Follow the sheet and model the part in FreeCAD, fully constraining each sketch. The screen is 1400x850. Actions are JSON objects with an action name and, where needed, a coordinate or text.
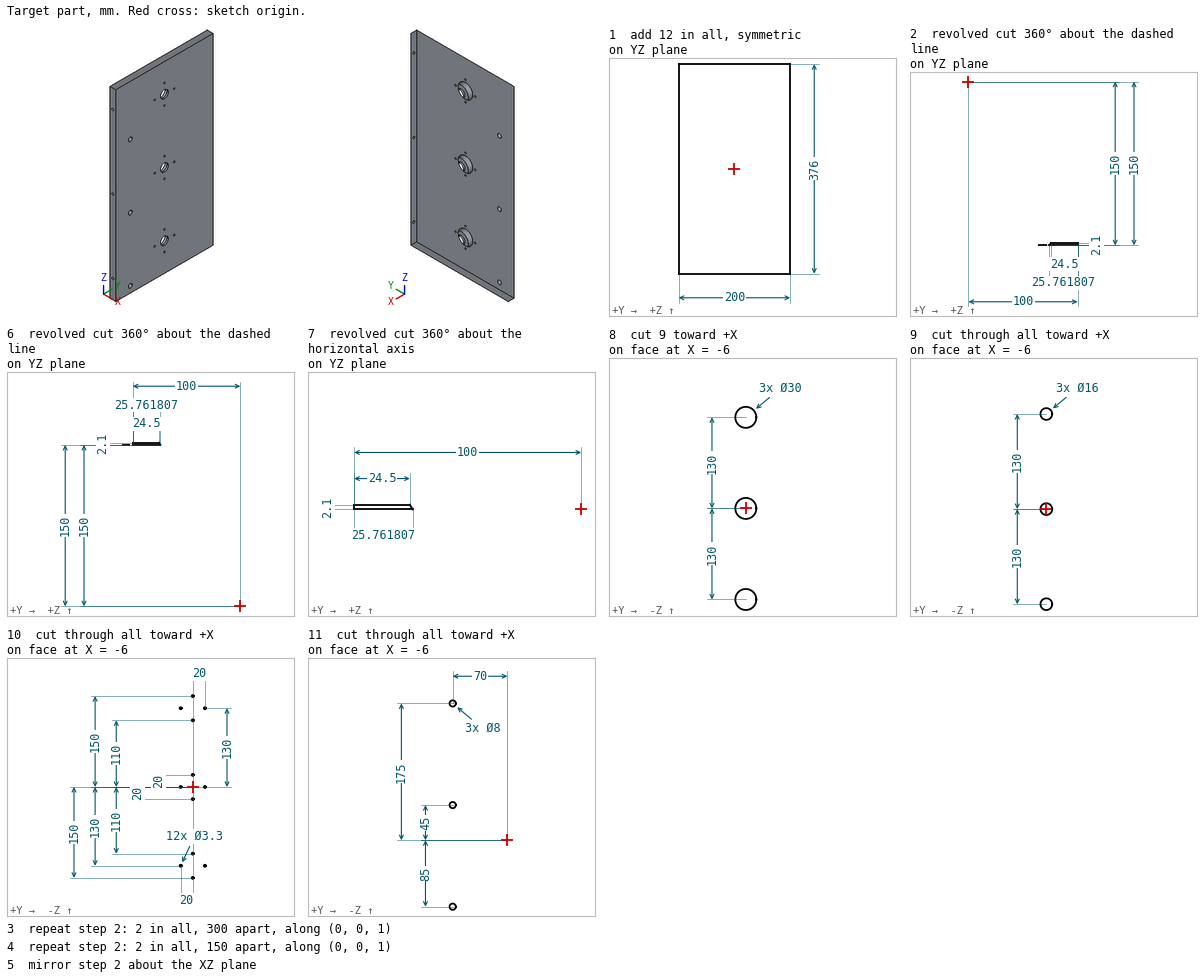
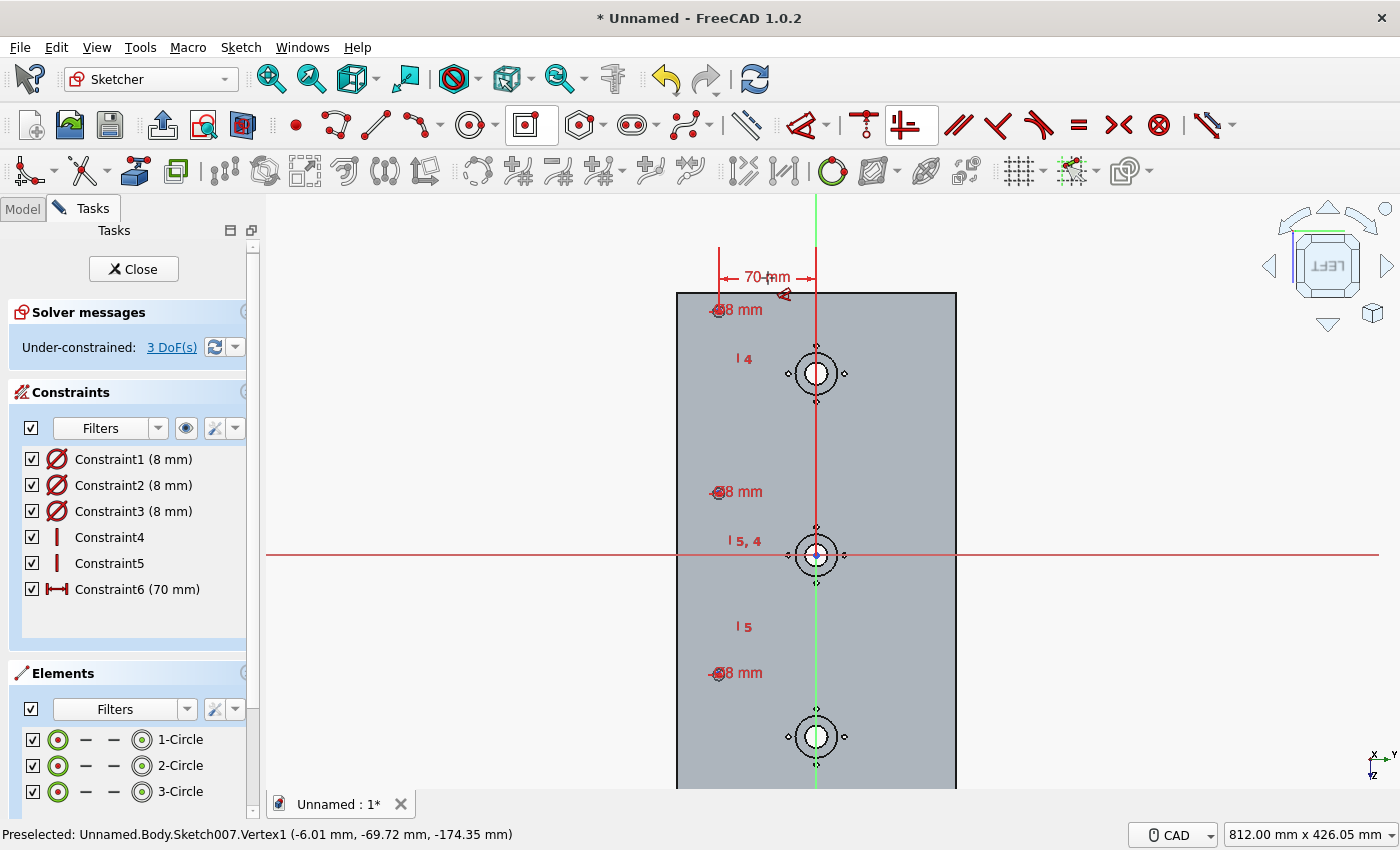
{"action": "left_click", "coordinate": [719, 494]}
{"action": "left_click", "coordinate": [850, 525]}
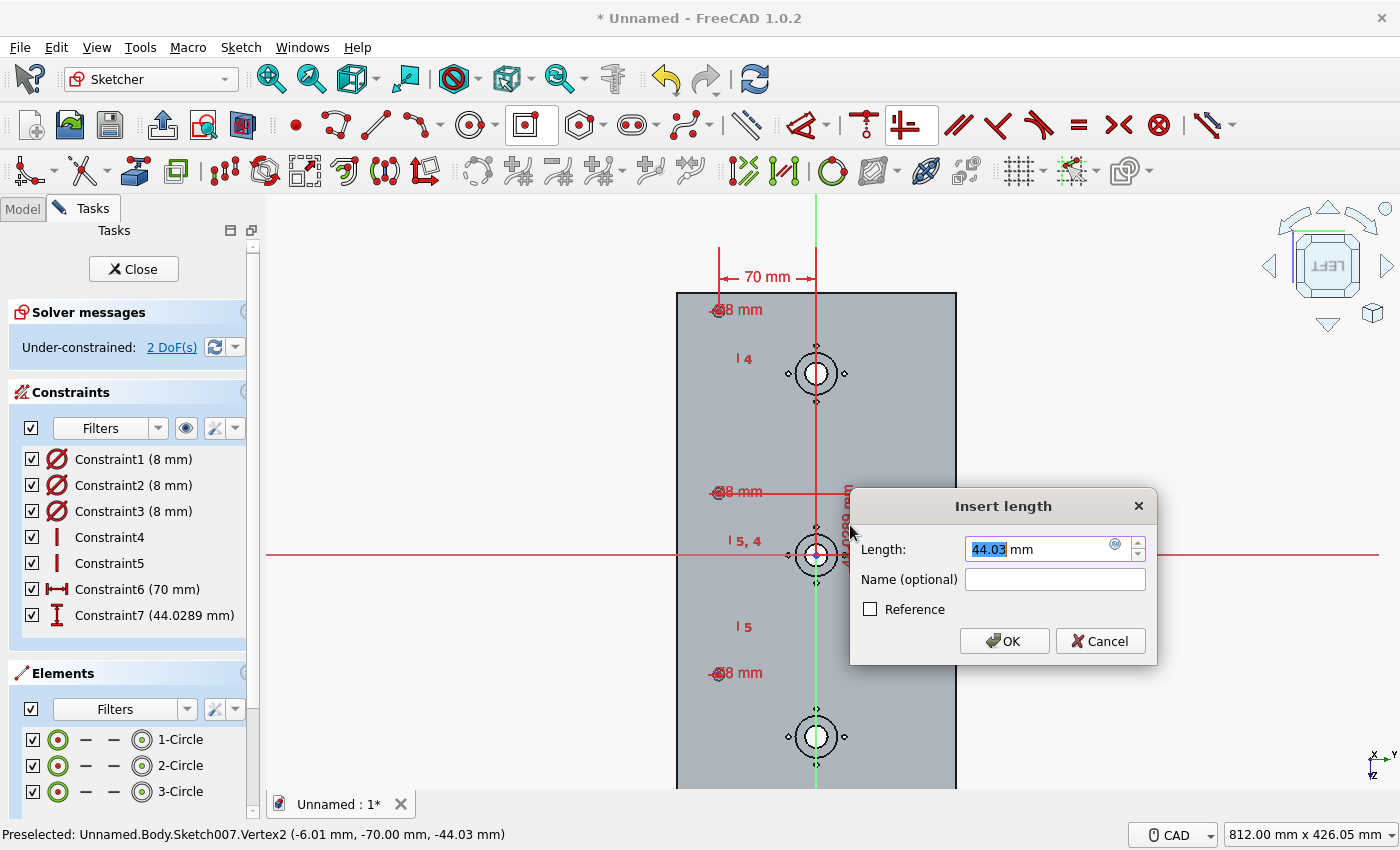
{"action": "type", "text": "45"}
{"action": "key", "text": "Return"}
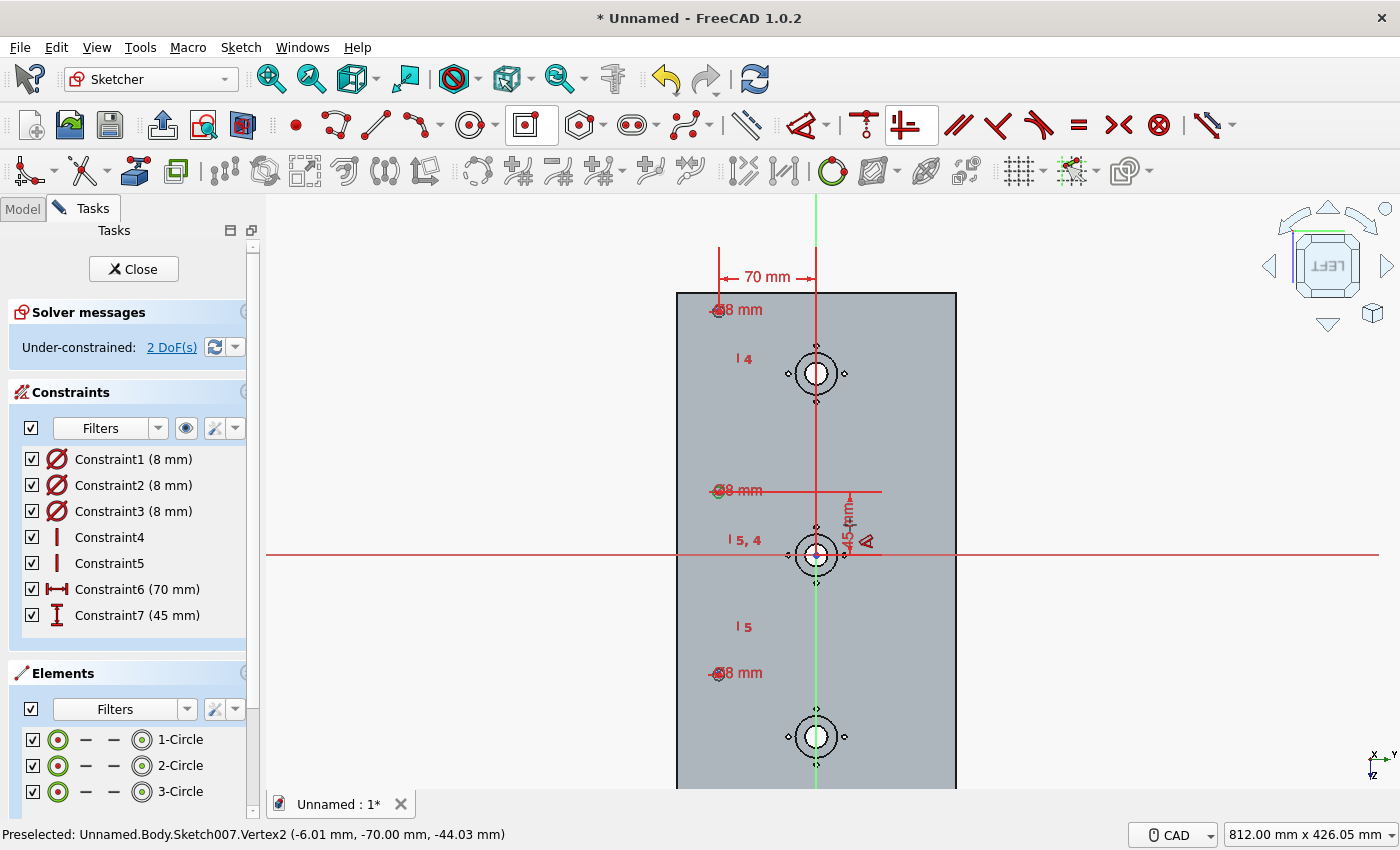
{"action": "left_click", "coordinate": [719, 675]}
{"action": "left_click", "coordinate": [850, 615]}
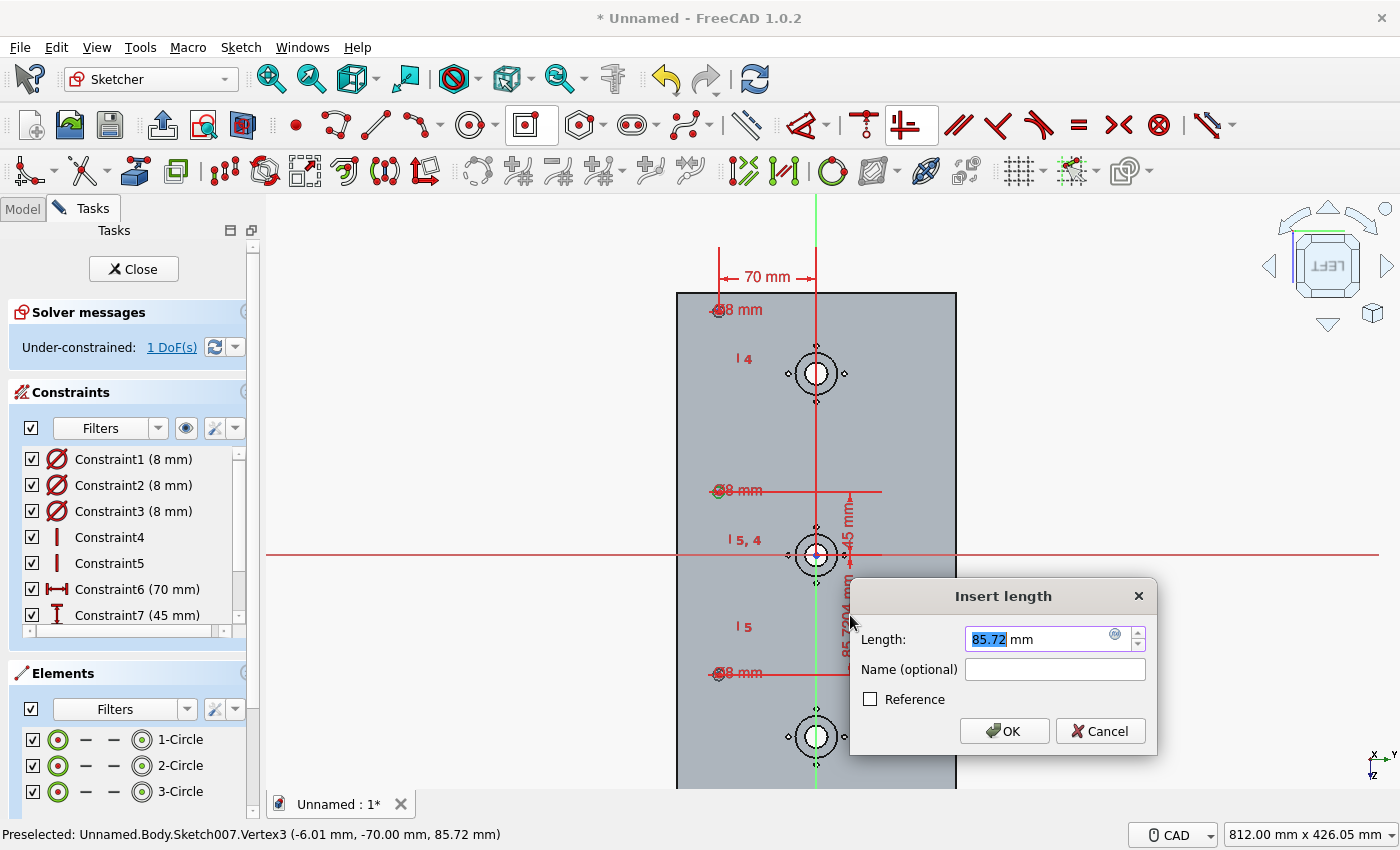
{"action": "type", "text": "85"}
{"action": "key", "text": "Return"}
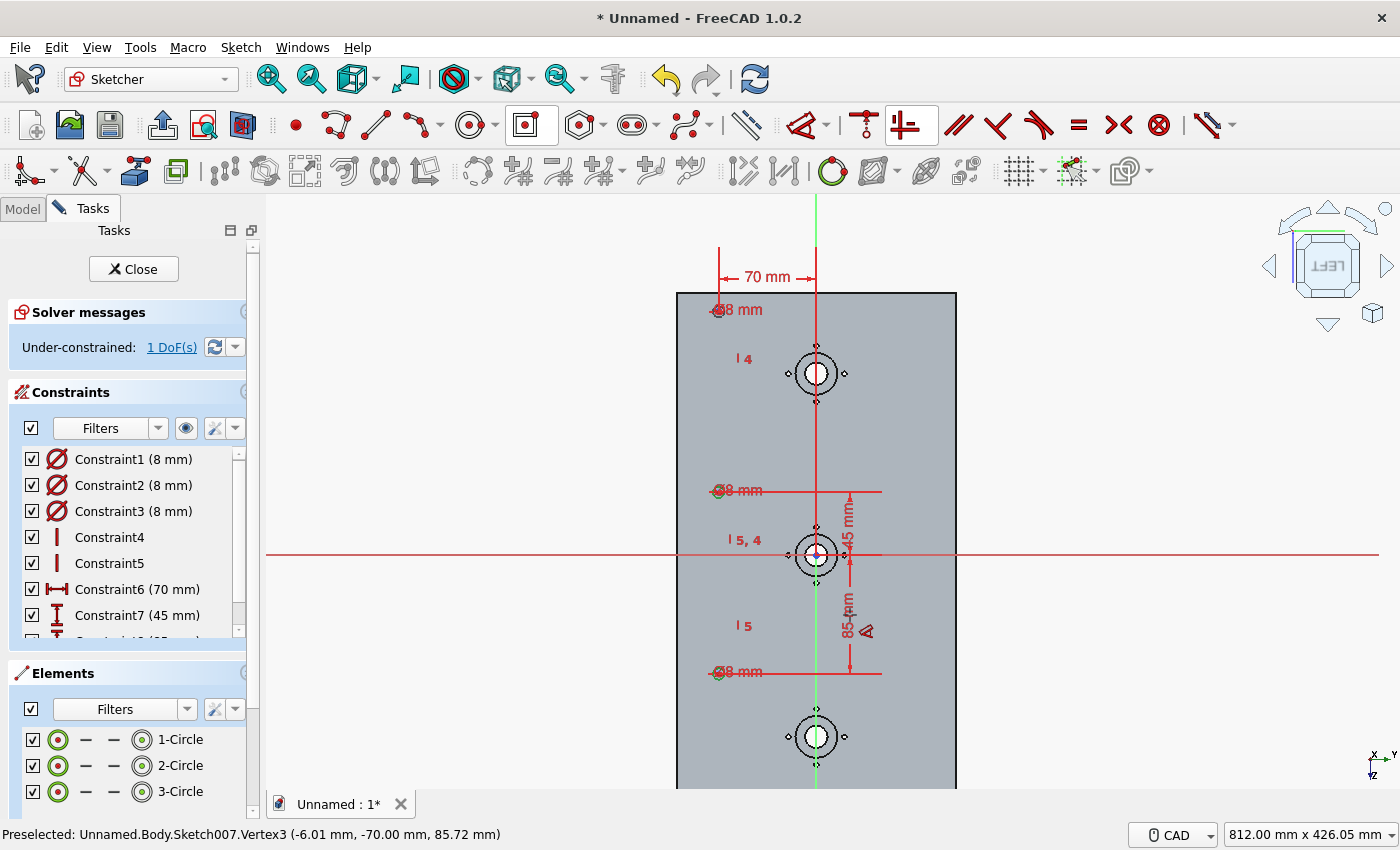
{"action": "left_click", "coordinate": [719, 312]}
{"action": "left_click", "coordinate": [850, 434]}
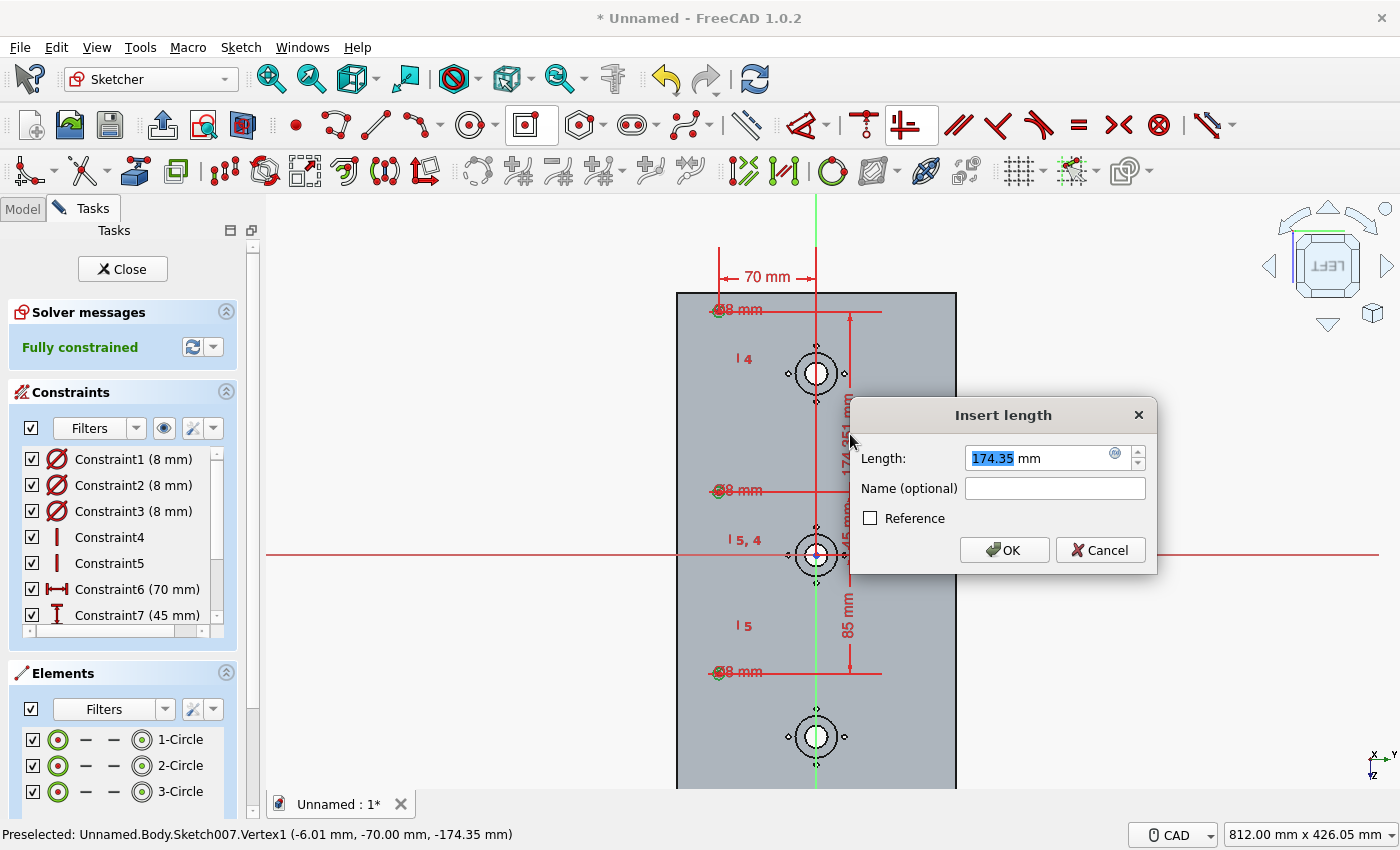
{"action": "type", "text": "175"}
{"action": "key", "text": "Return"}
{"action": "key", "text": "Escape"}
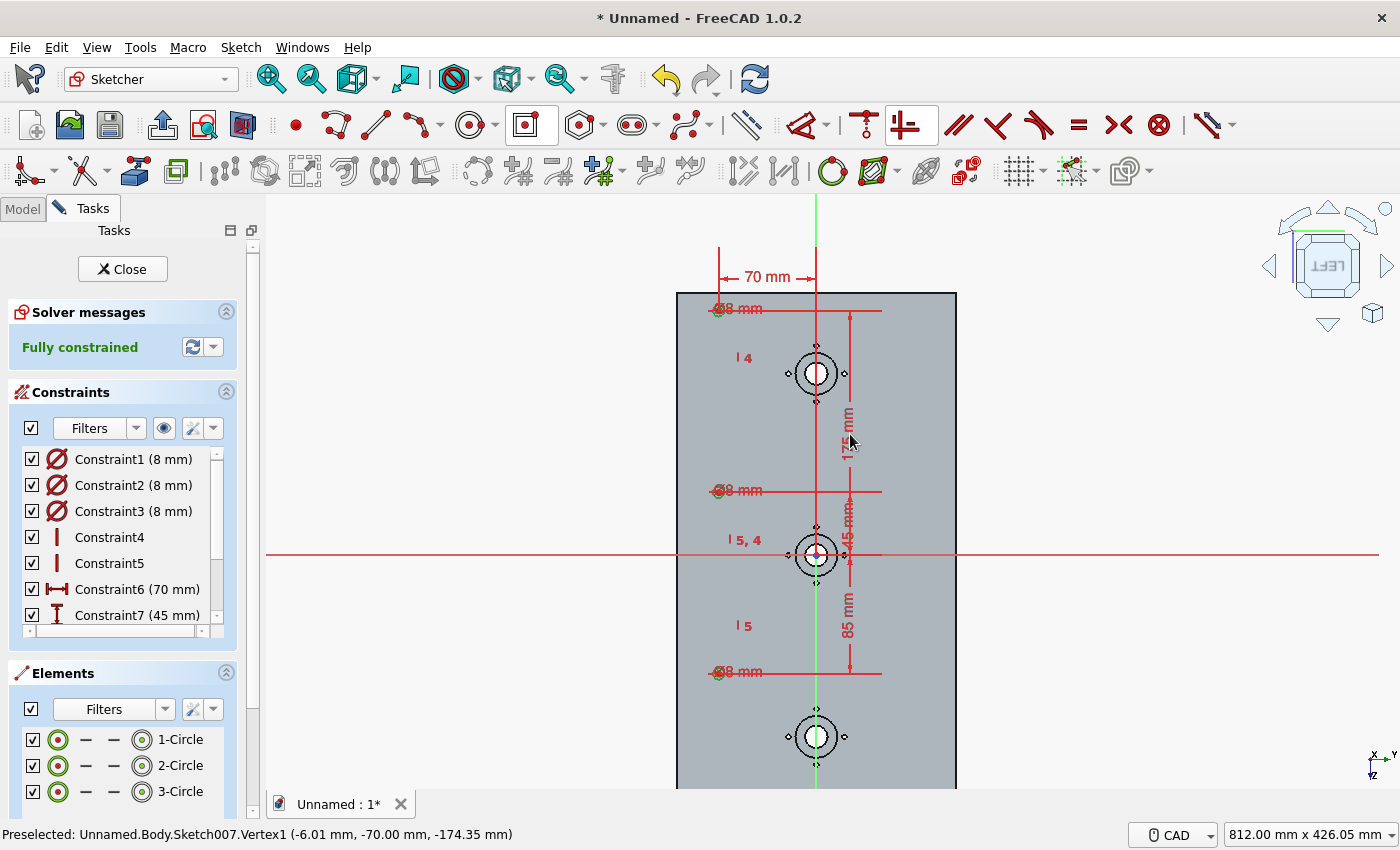
{"action": "left_click", "coordinate": [123, 269]}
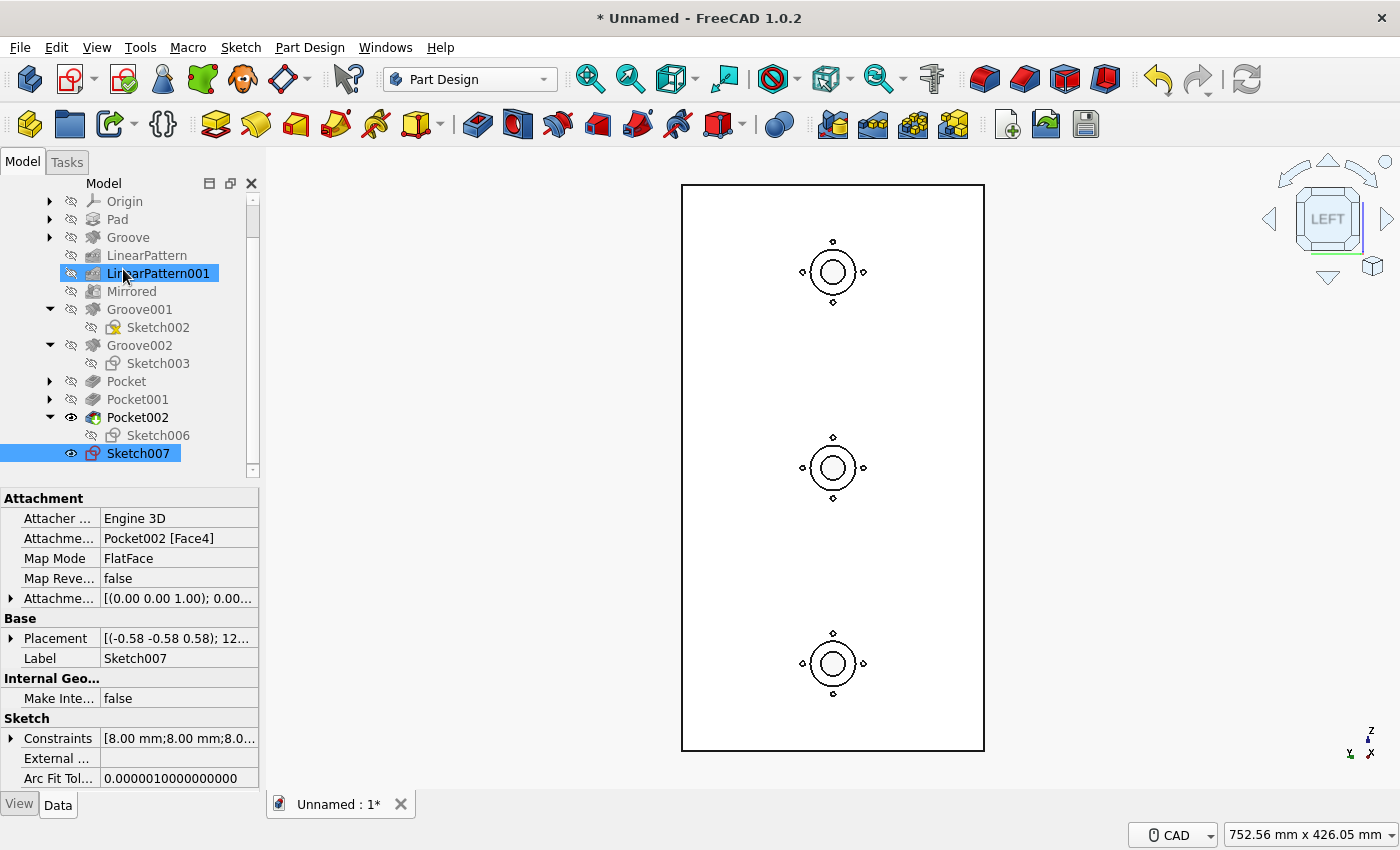
{"action": "left_click", "coordinate": [478, 124]}